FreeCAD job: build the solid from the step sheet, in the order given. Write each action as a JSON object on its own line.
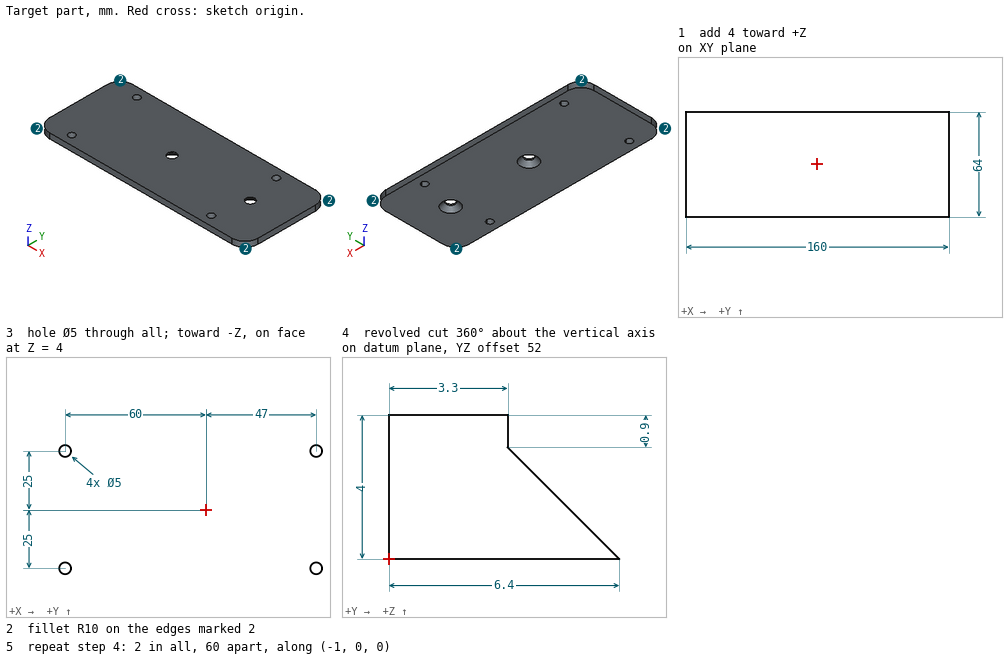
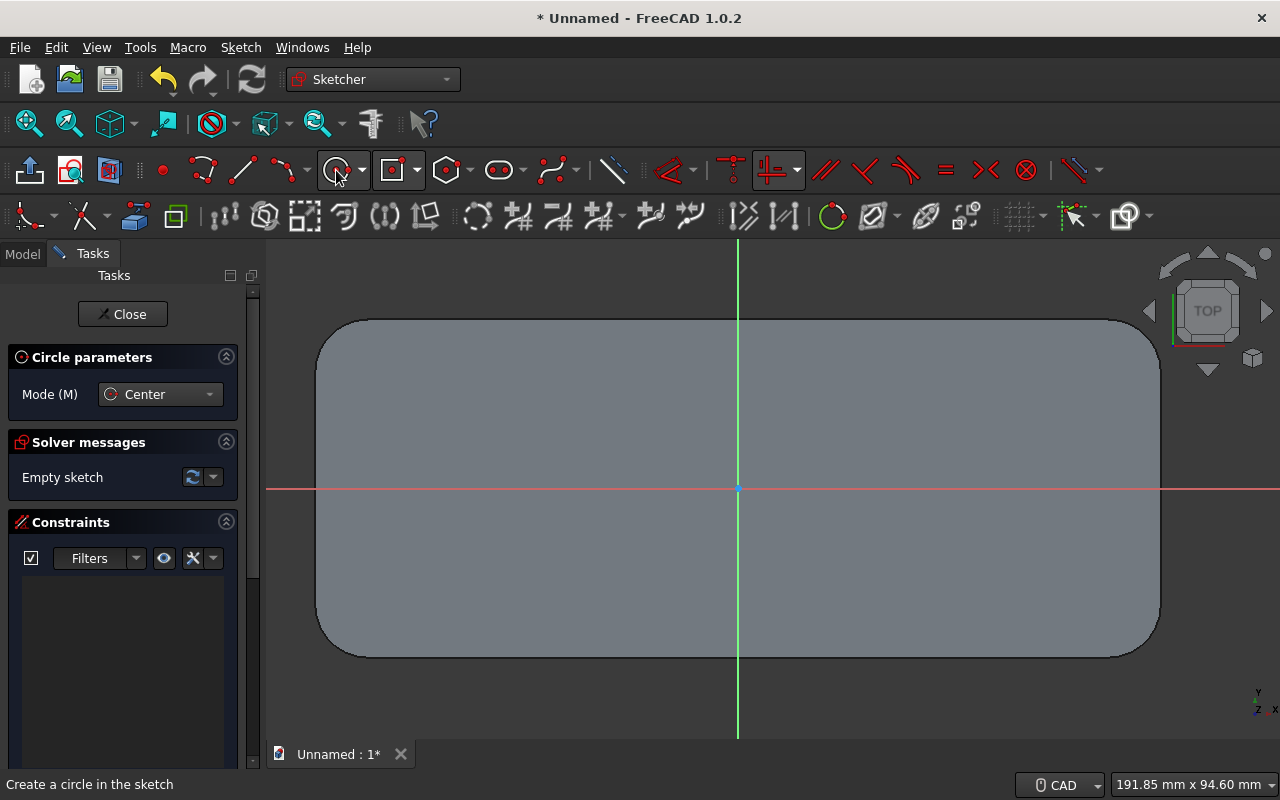
{"action": "scroll", "coordinate": [421, 356], "scroll_direction": "up", "scroll_amount": 3}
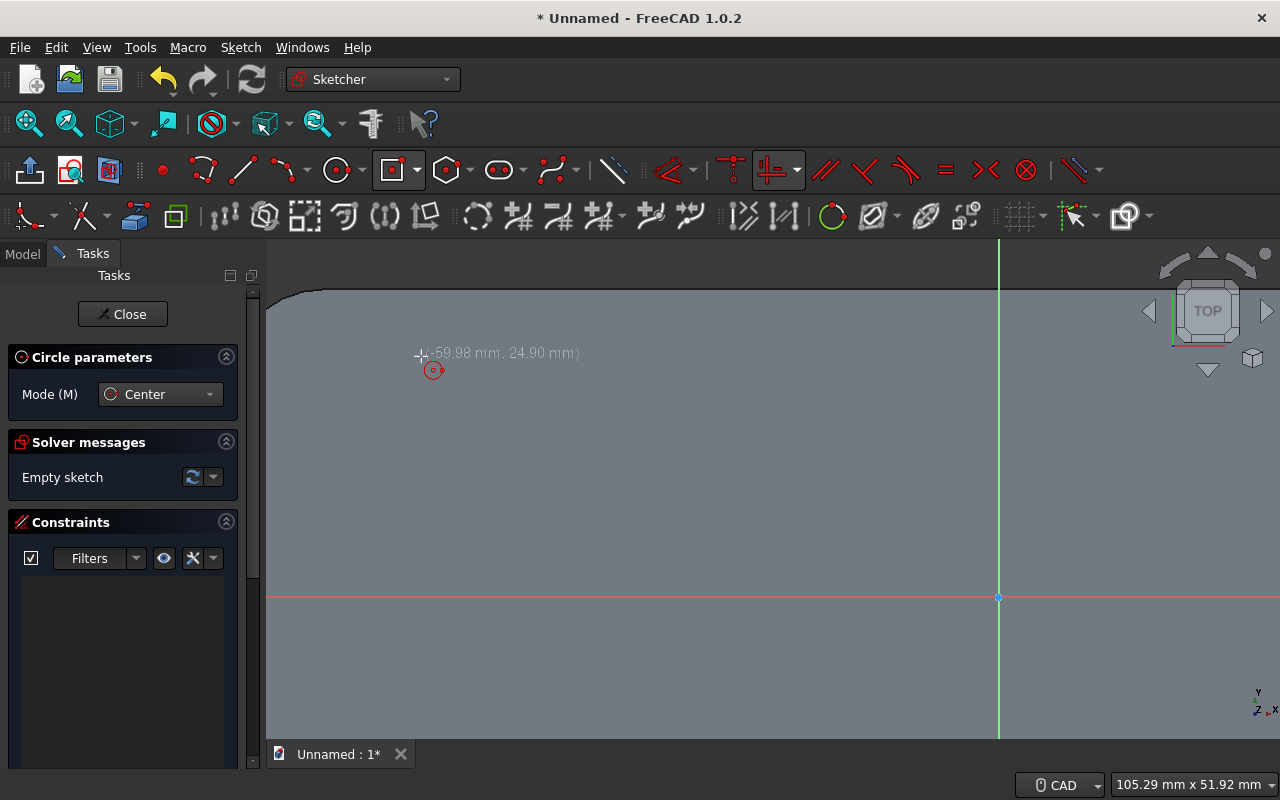
{"action": "left_click", "coordinate": [421, 357]}
{"action": "left_click", "coordinate": [438, 340]}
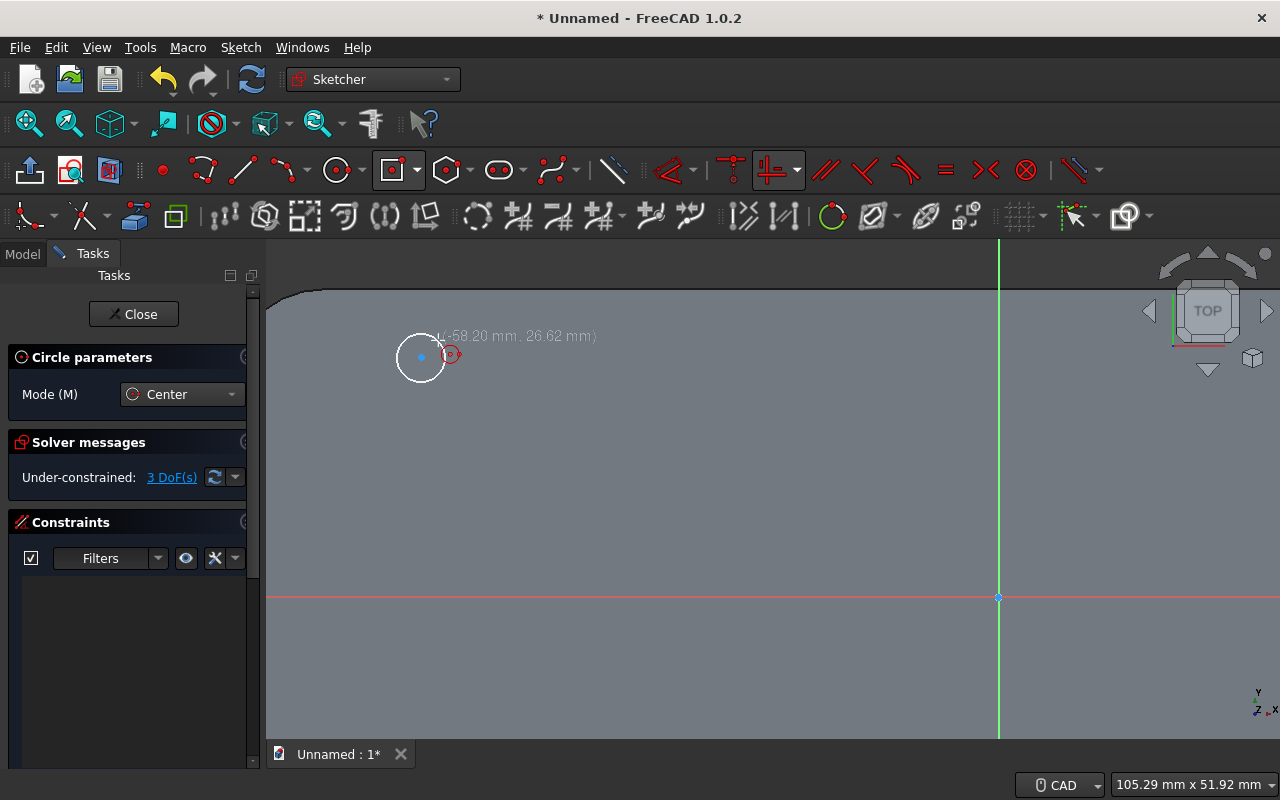
{"action": "scroll", "coordinate": [423, 357], "scroll_direction": "down", "scroll_amount": 3}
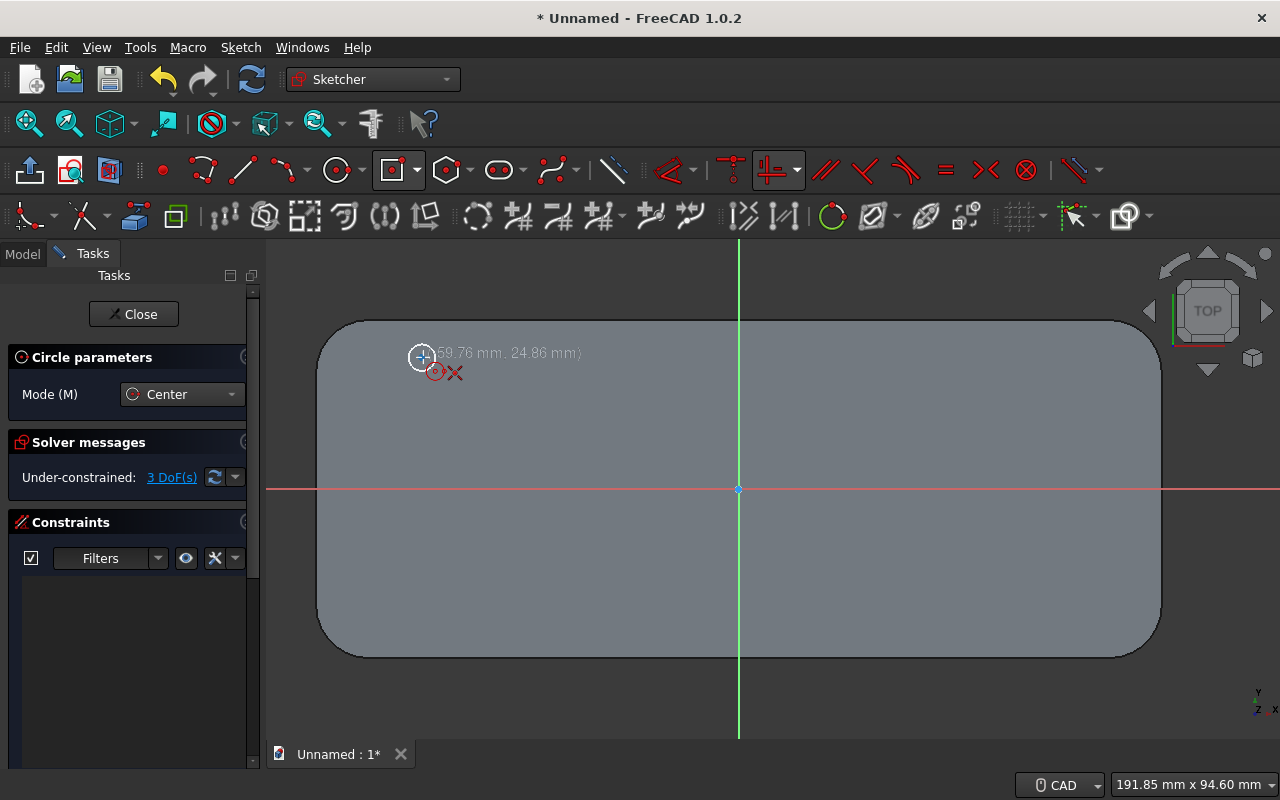
{"action": "scroll", "coordinate": [422, 621], "scroll_direction": "up", "scroll_amount": 3}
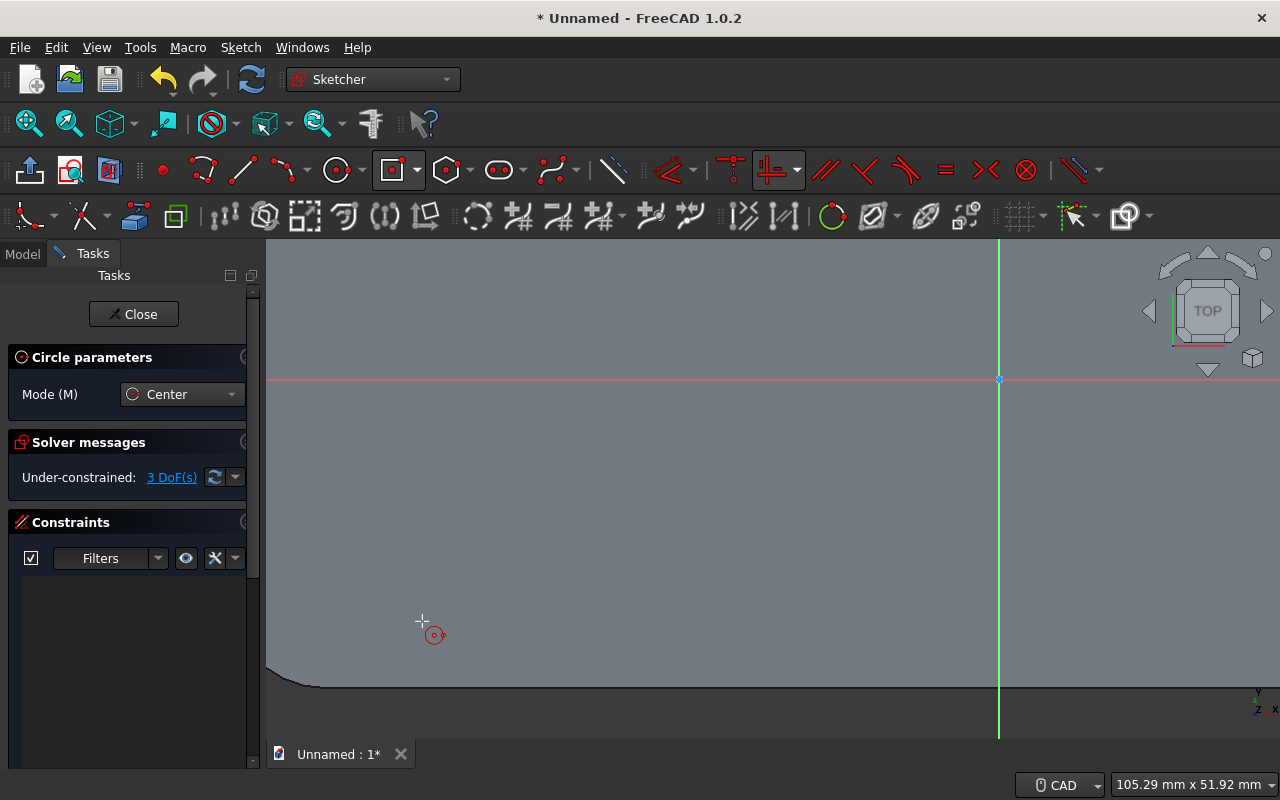
{"action": "left_click", "coordinate": [422, 621]}
{"action": "left_click", "coordinate": [439, 604]}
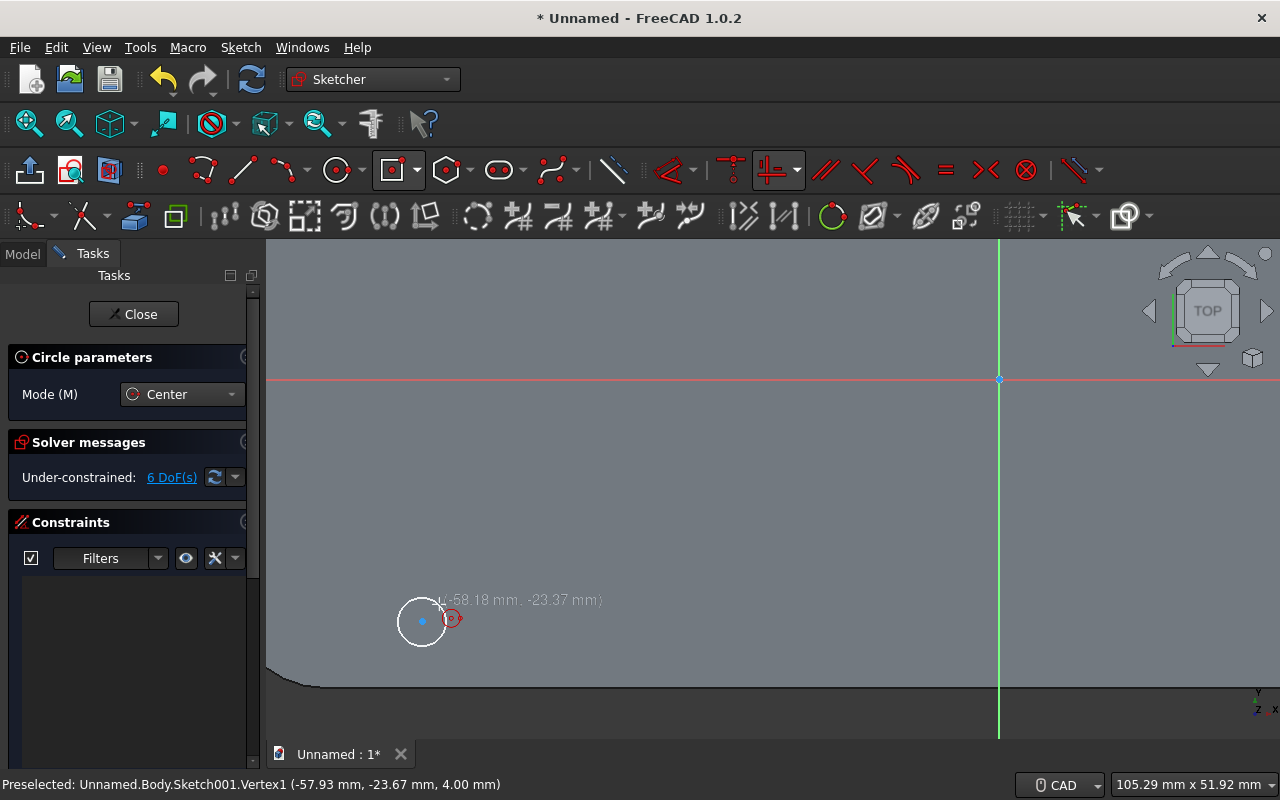
{"action": "scroll", "coordinate": [422, 622], "scroll_direction": "down", "scroll_amount": 3}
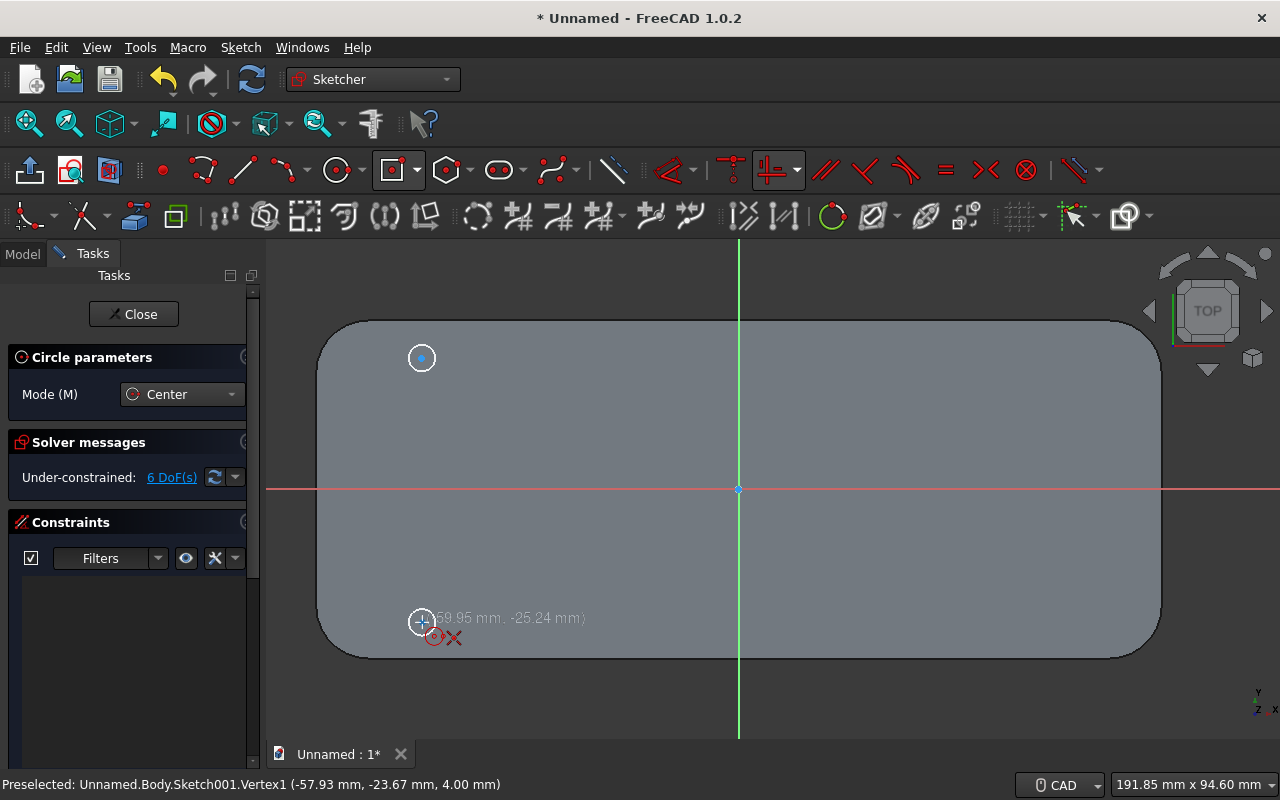
{"action": "scroll", "coordinate": [987, 357], "scroll_direction": "up", "scroll_amount": 3}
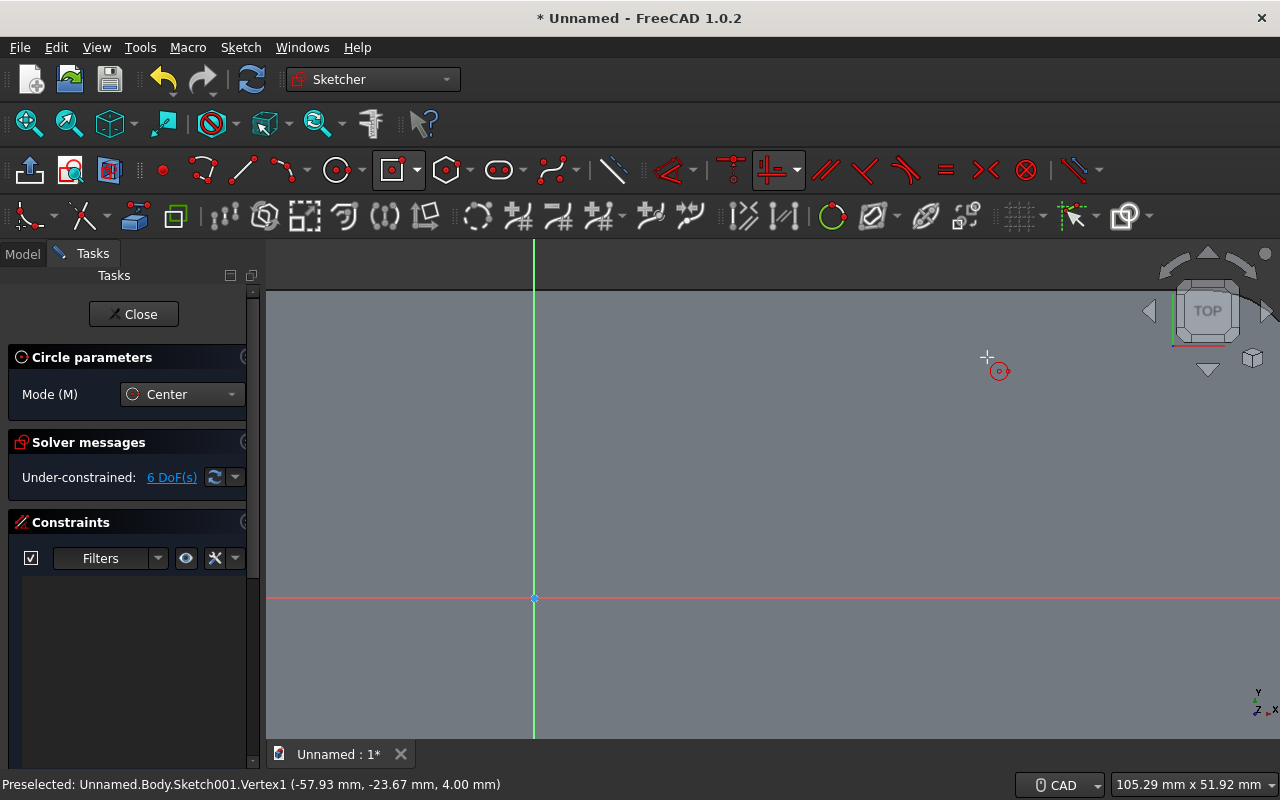
{"action": "left_click", "coordinate": [987, 357]}
{"action": "left_click", "coordinate": [1004, 340]}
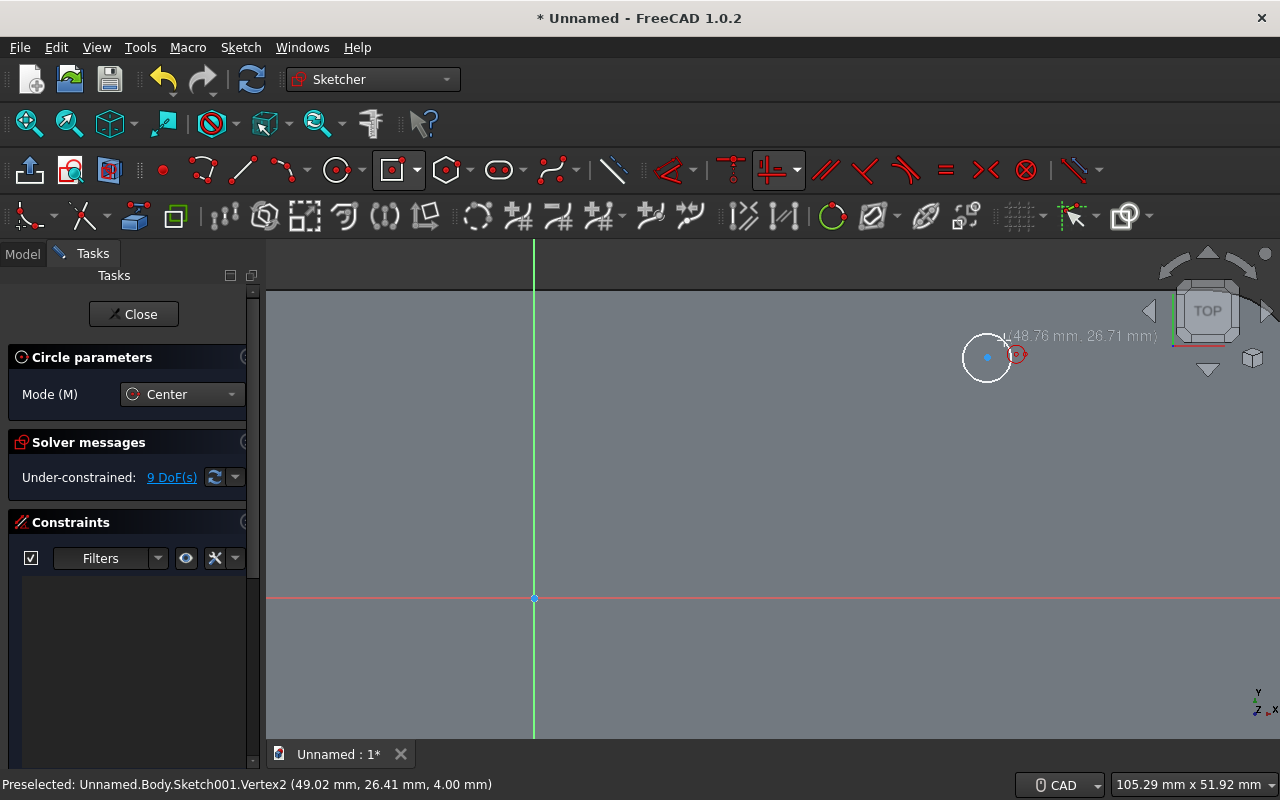
{"action": "scroll", "coordinate": [988, 356], "scroll_direction": "down", "scroll_amount": 3}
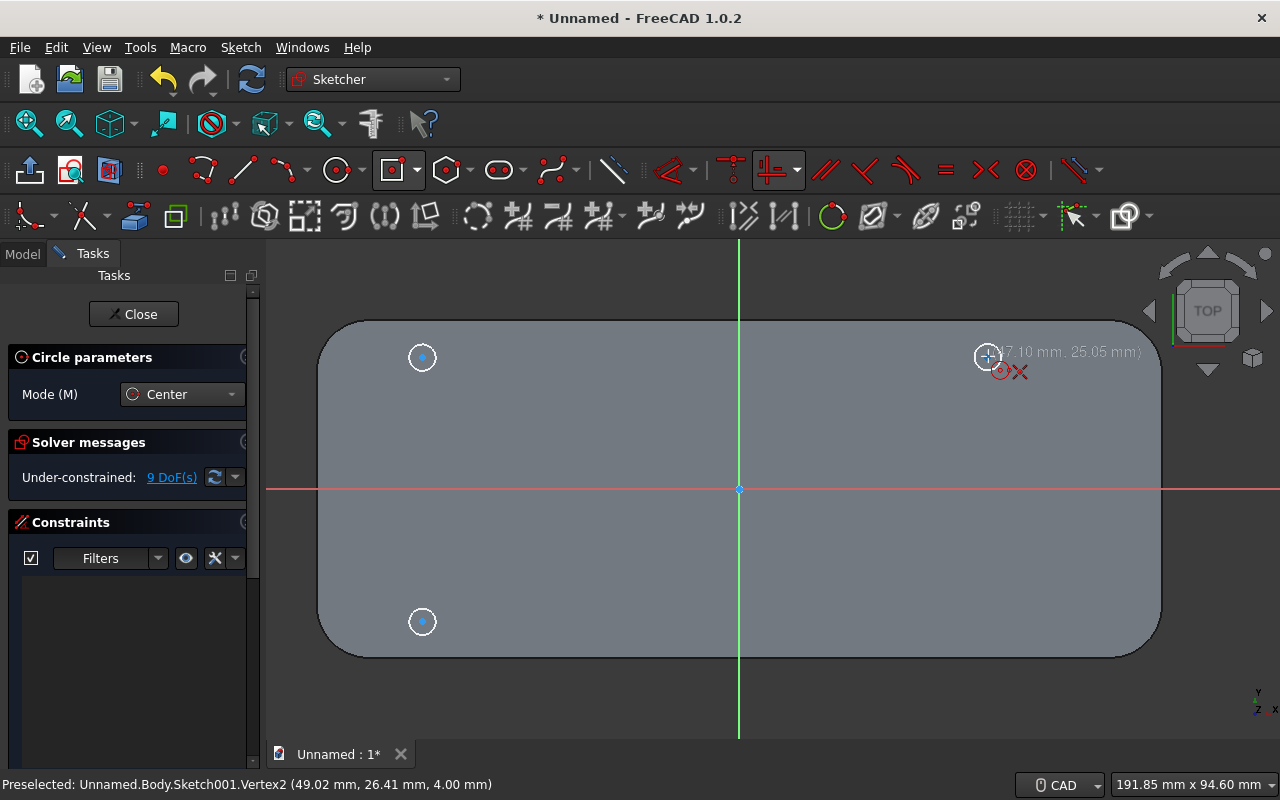
{"action": "scroll", "coordinate": [988, 621], "scroll_direction": "up", "scroll_amount": 3}